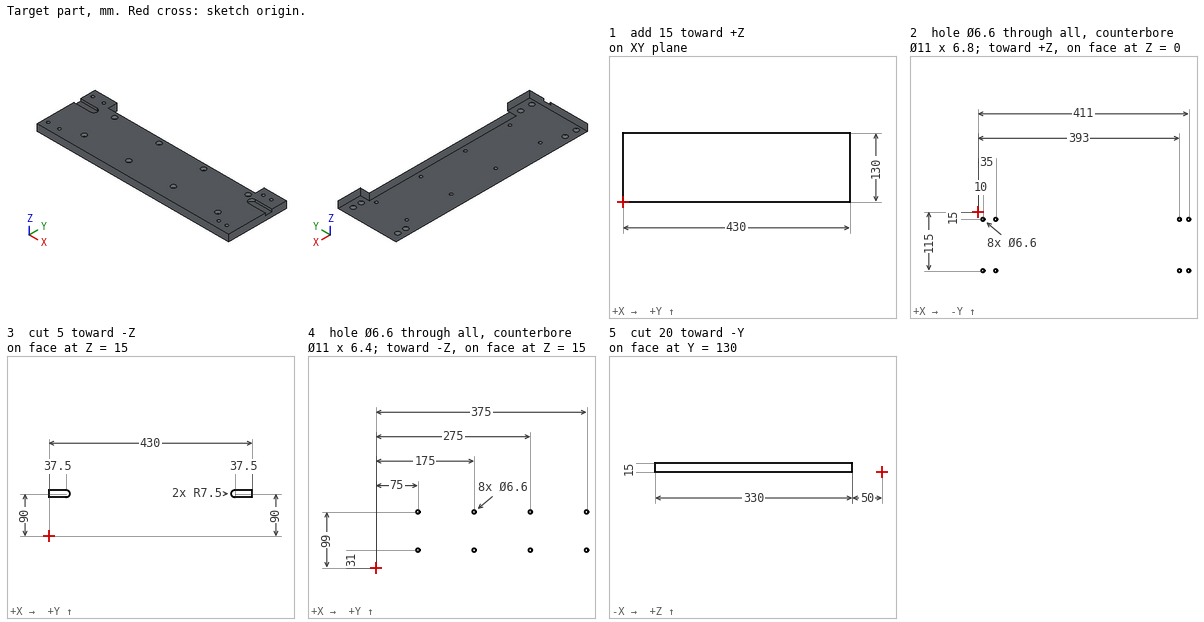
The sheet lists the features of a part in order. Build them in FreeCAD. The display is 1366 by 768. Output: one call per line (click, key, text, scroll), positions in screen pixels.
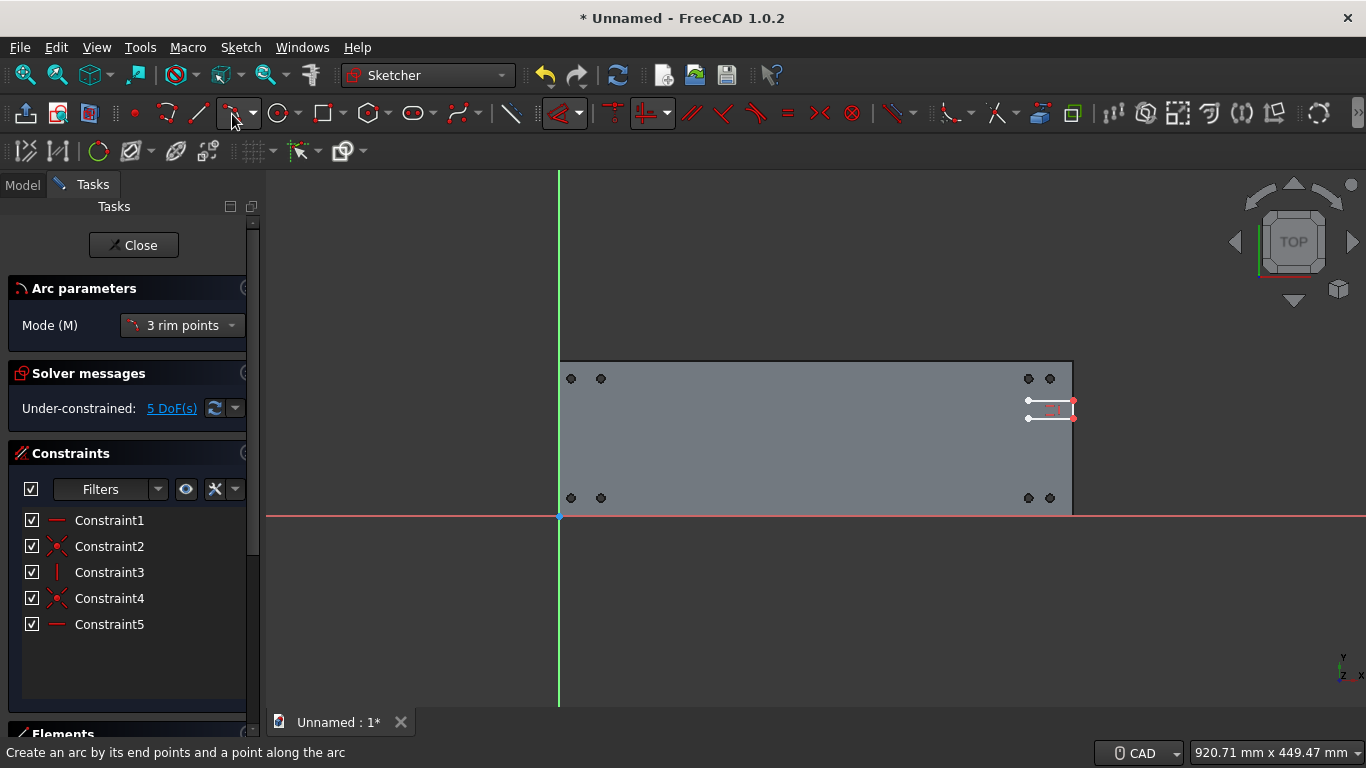
click(1028, 401)
click(1028, 419)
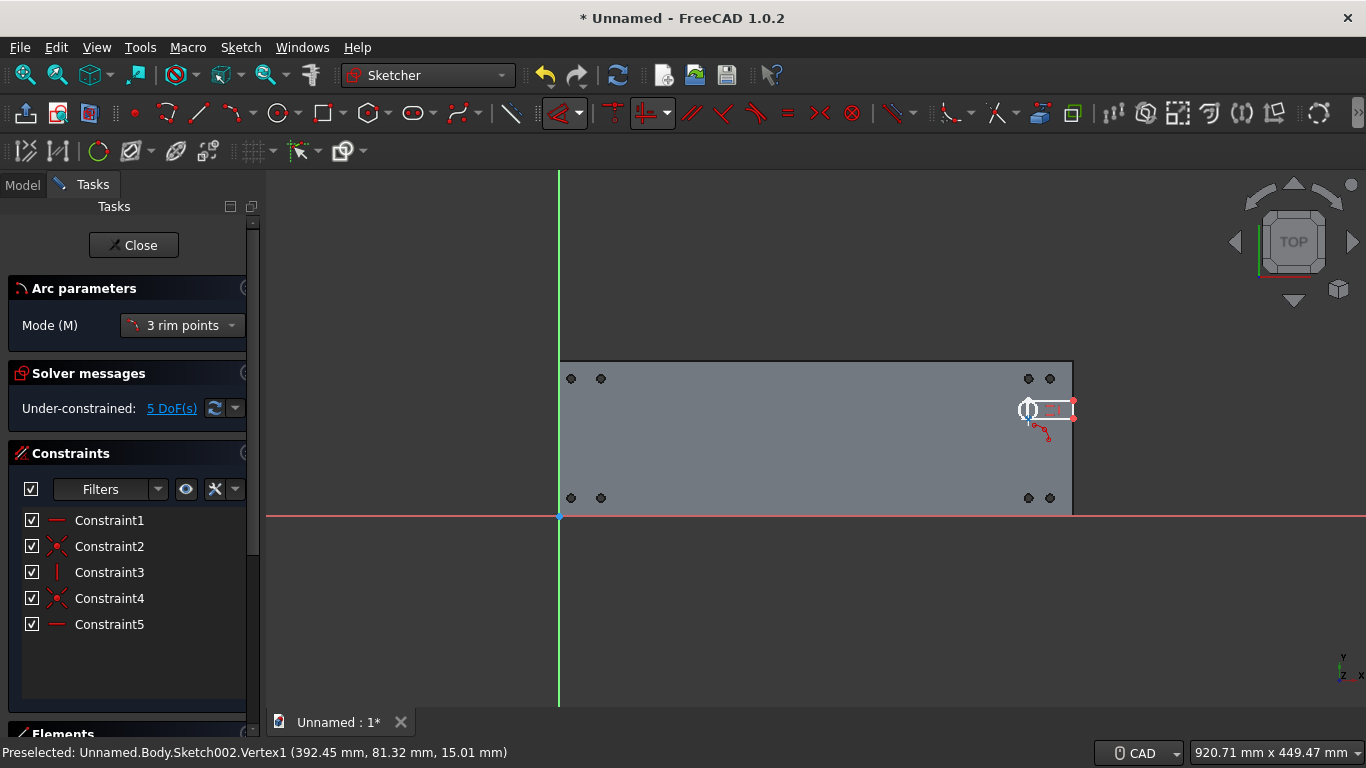
scroll(1019, 409, up, 3)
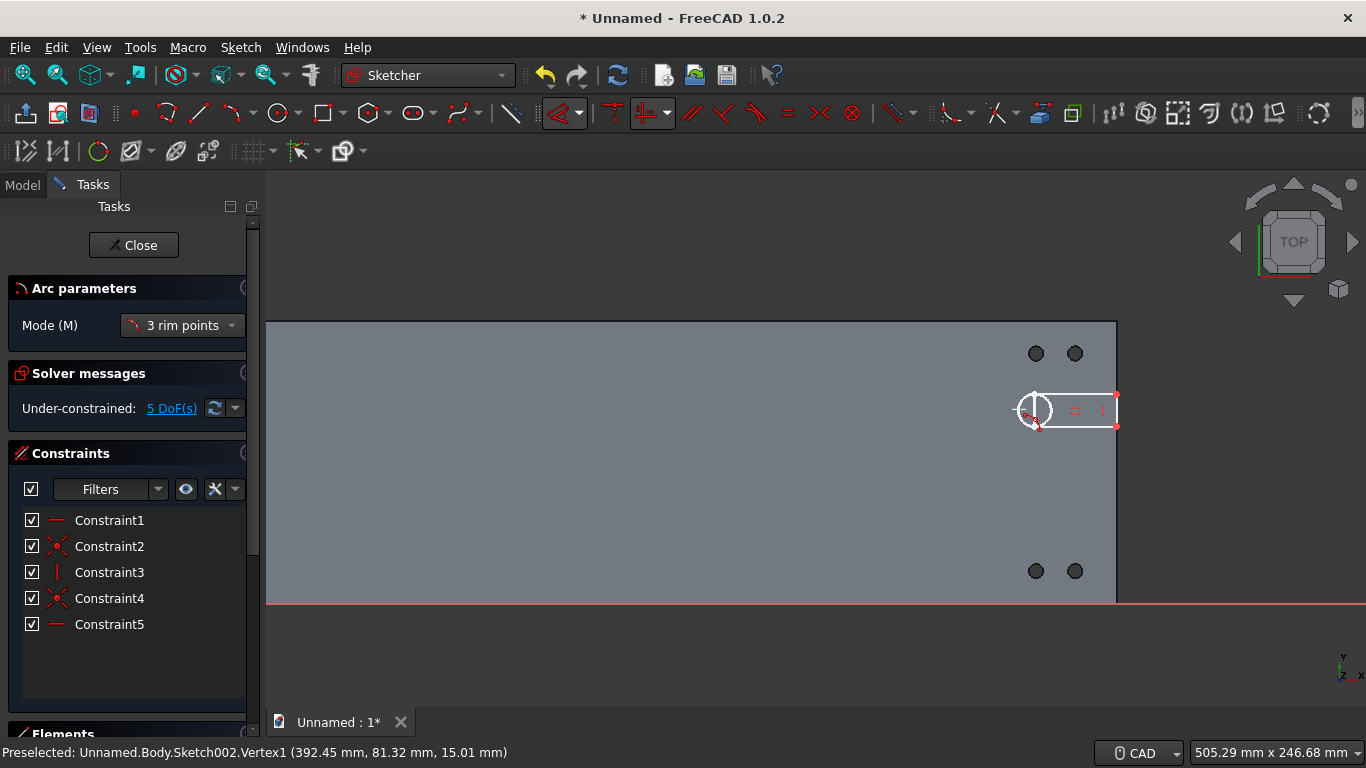
click(1019, 408)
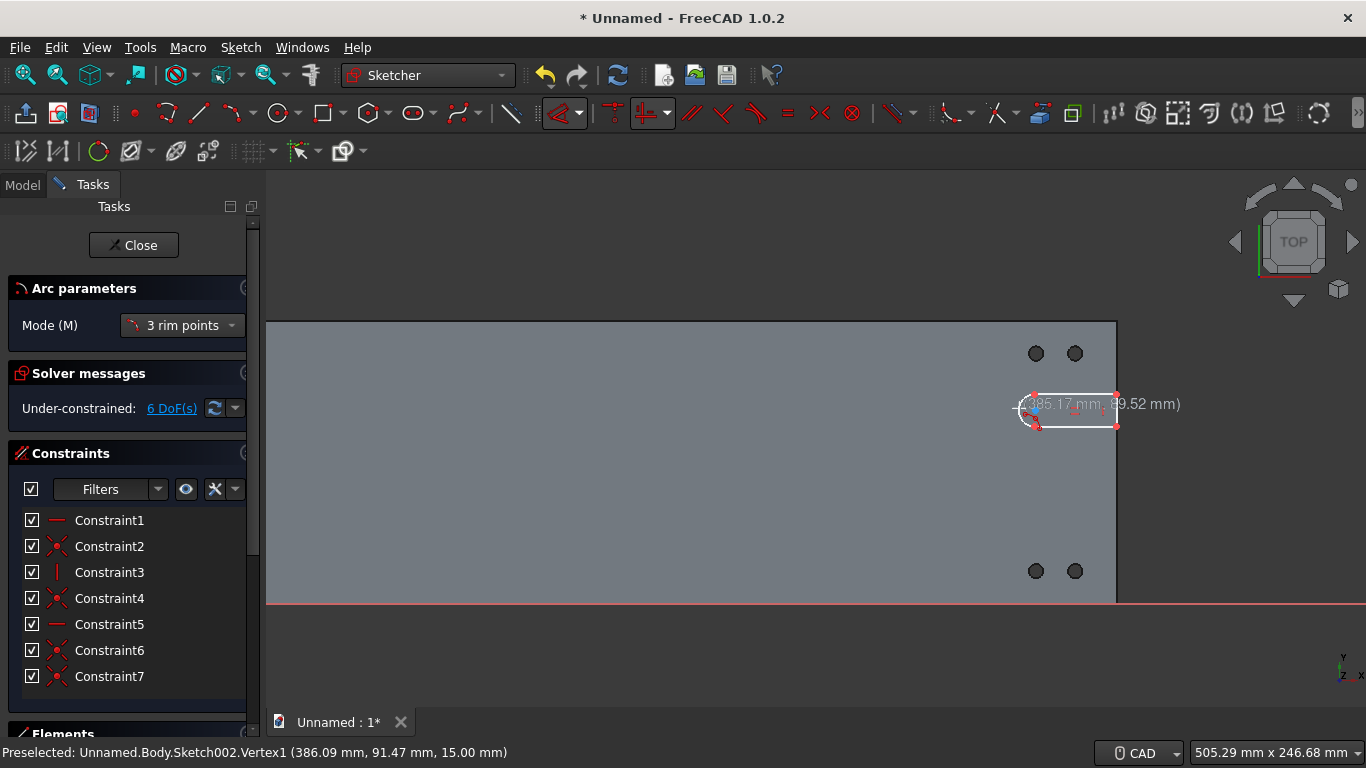
click(168, 114)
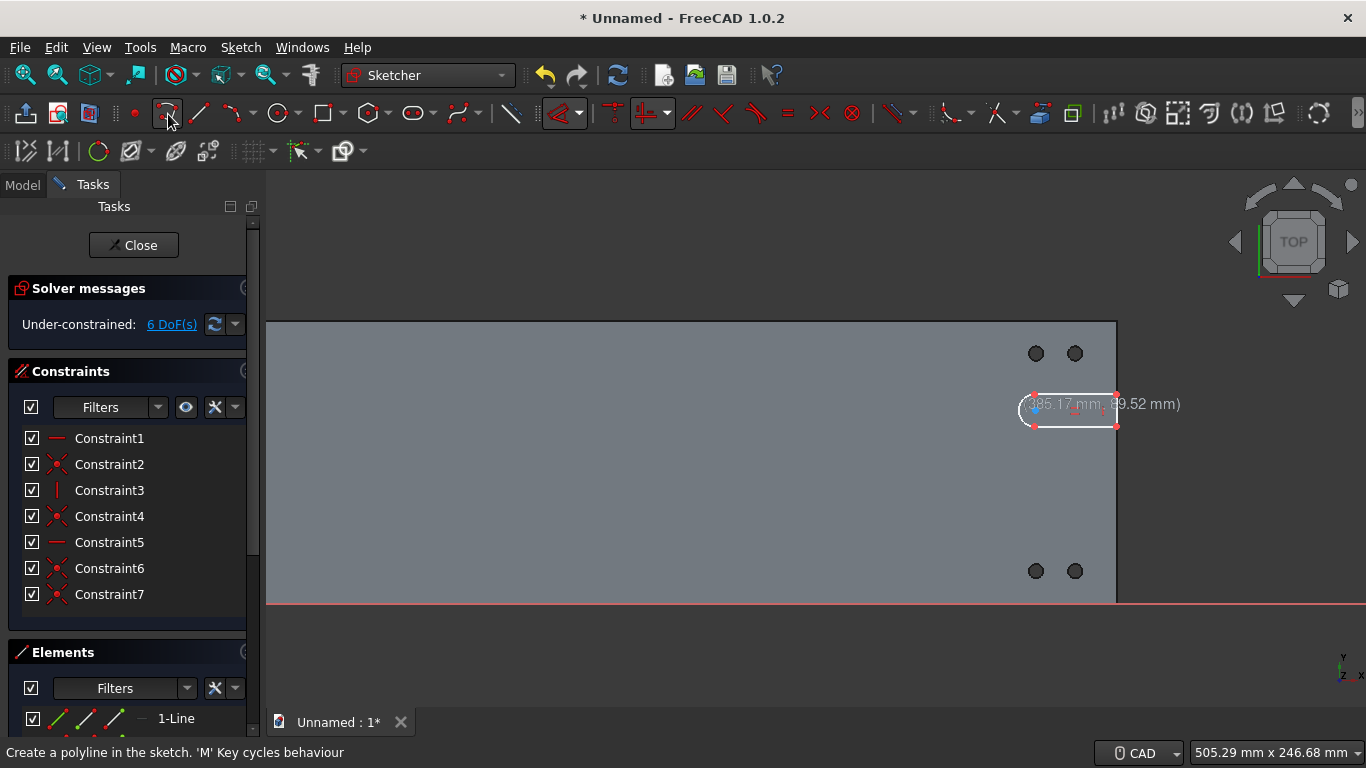
scroll(949, 318, down, 2)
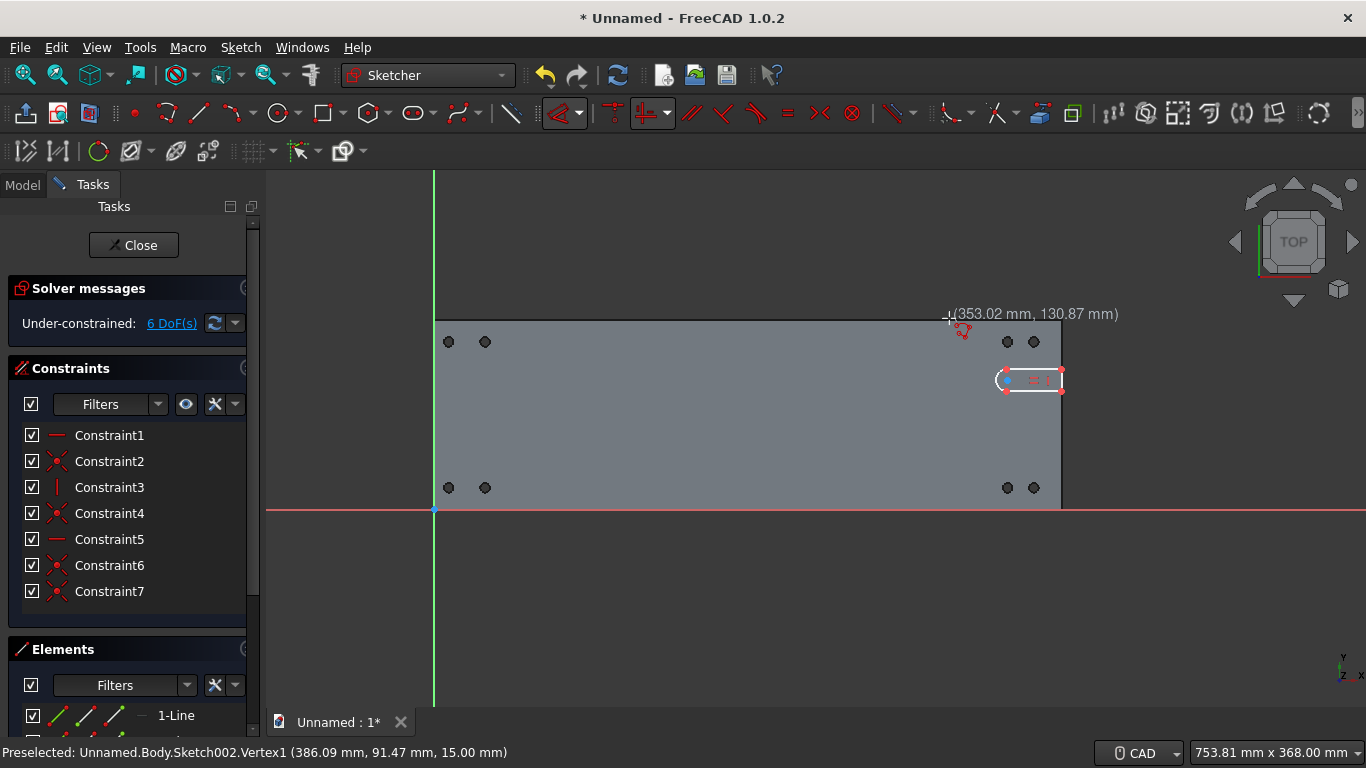
click(489, 367)
click(434, 367)
click(443, 389)
click(489, 389)
right_click(489, 389)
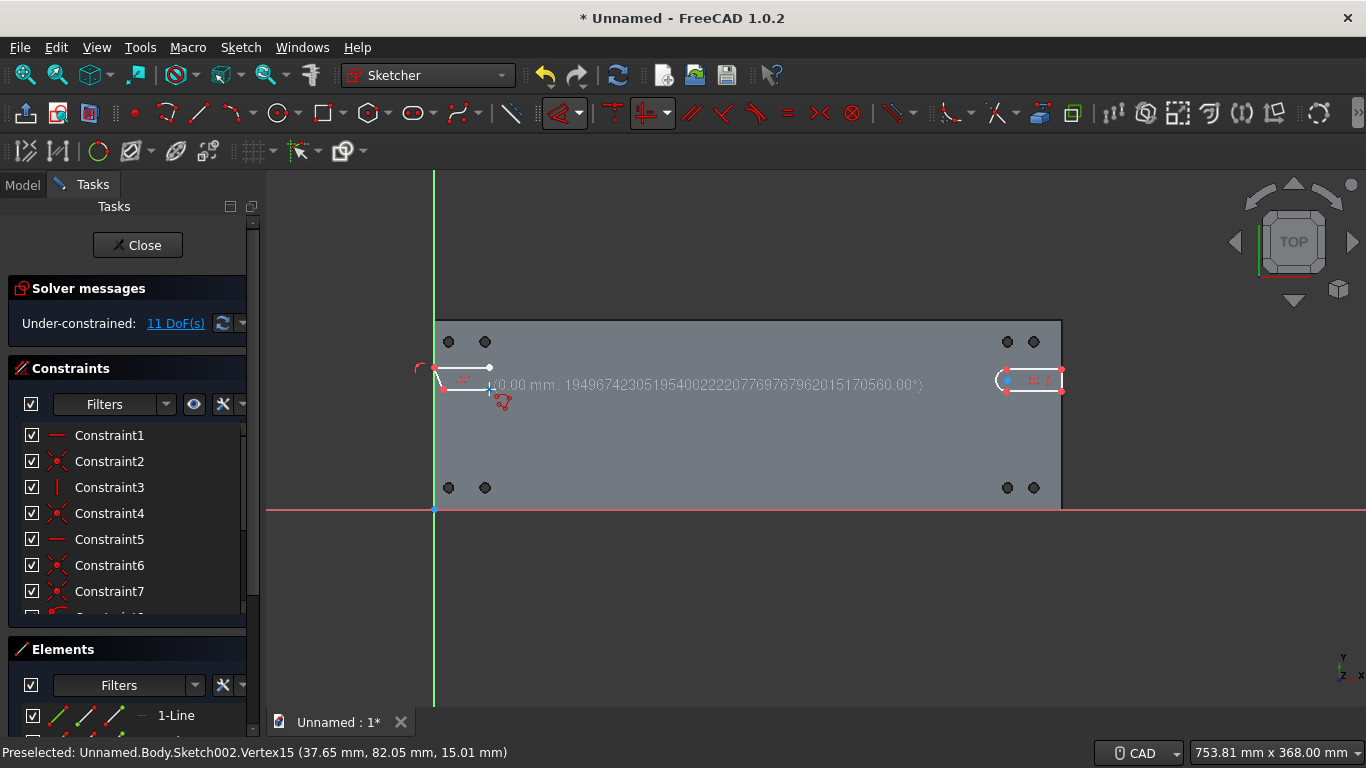
key(g)
key(3)
key(a)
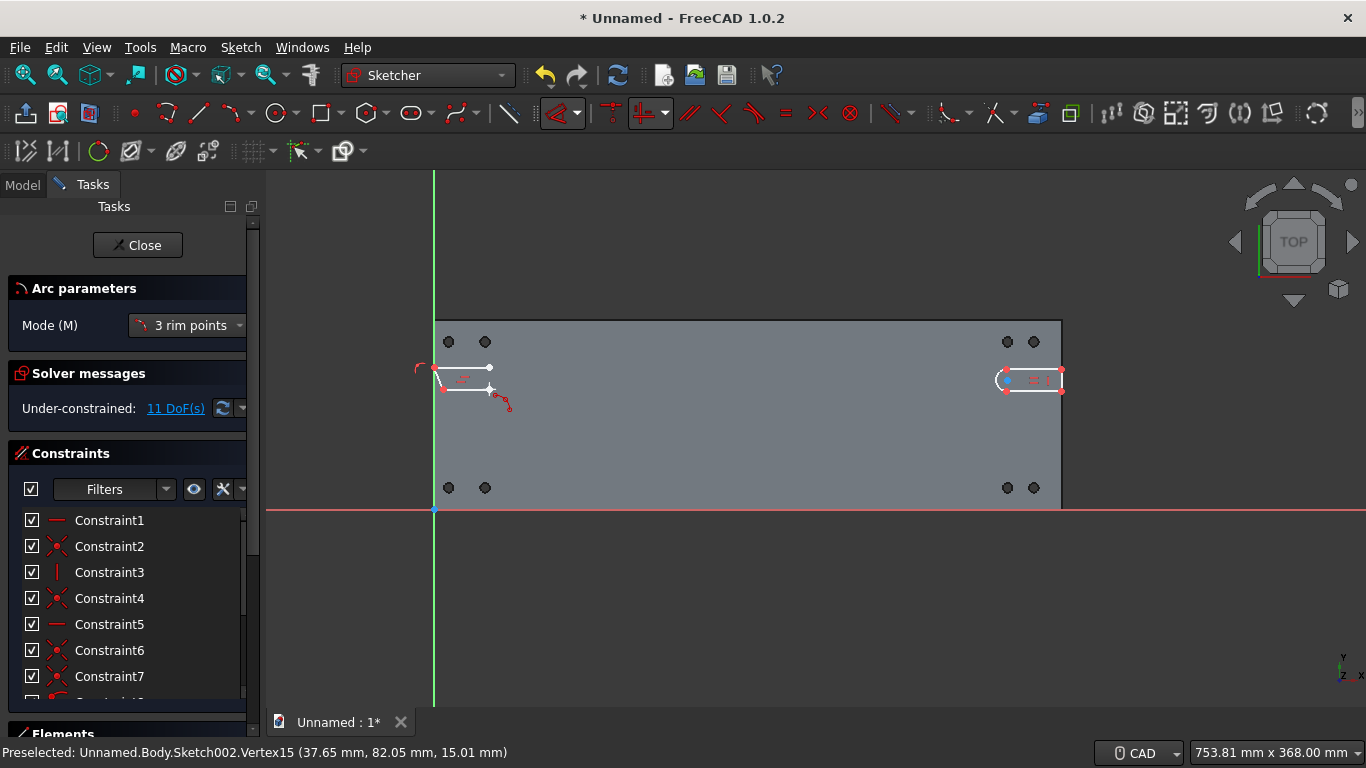
click(489, 390)
click(489, 368)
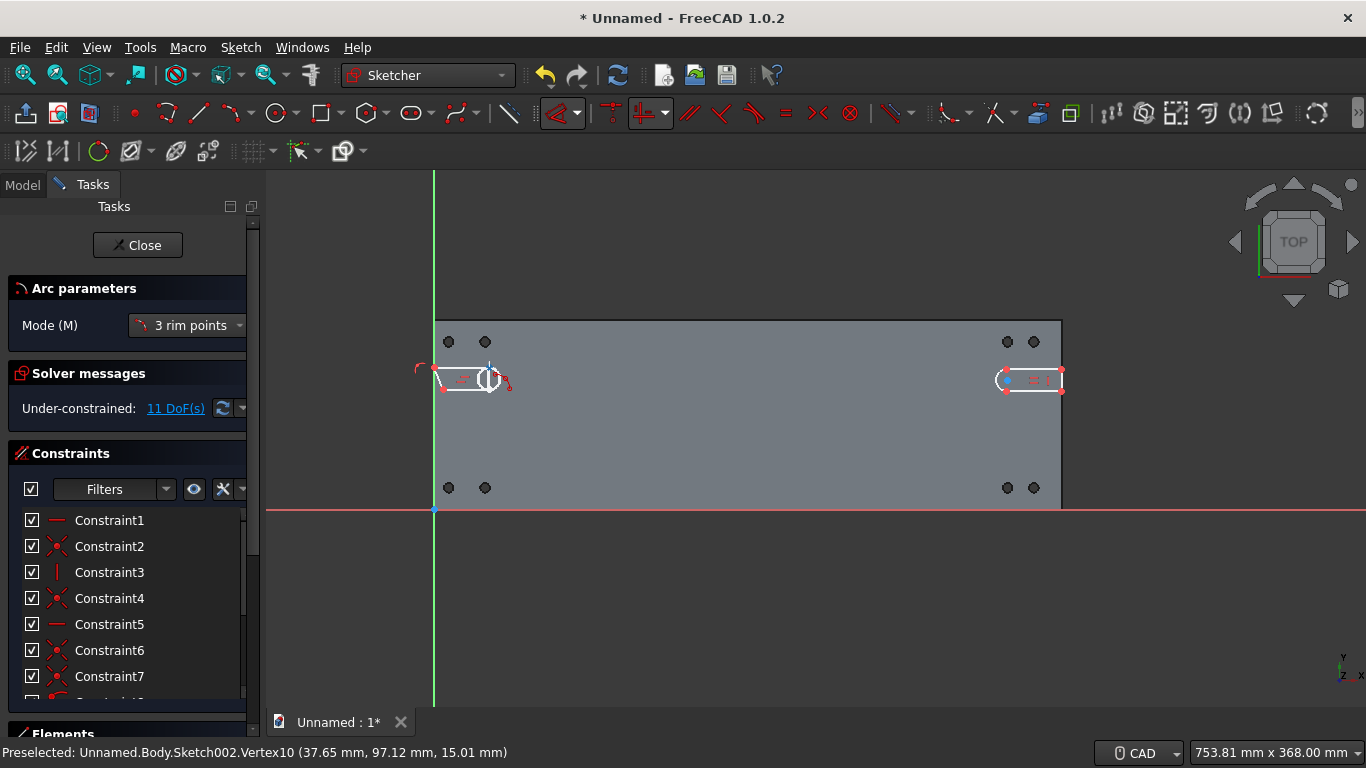
scroll(500, 378, up, 2)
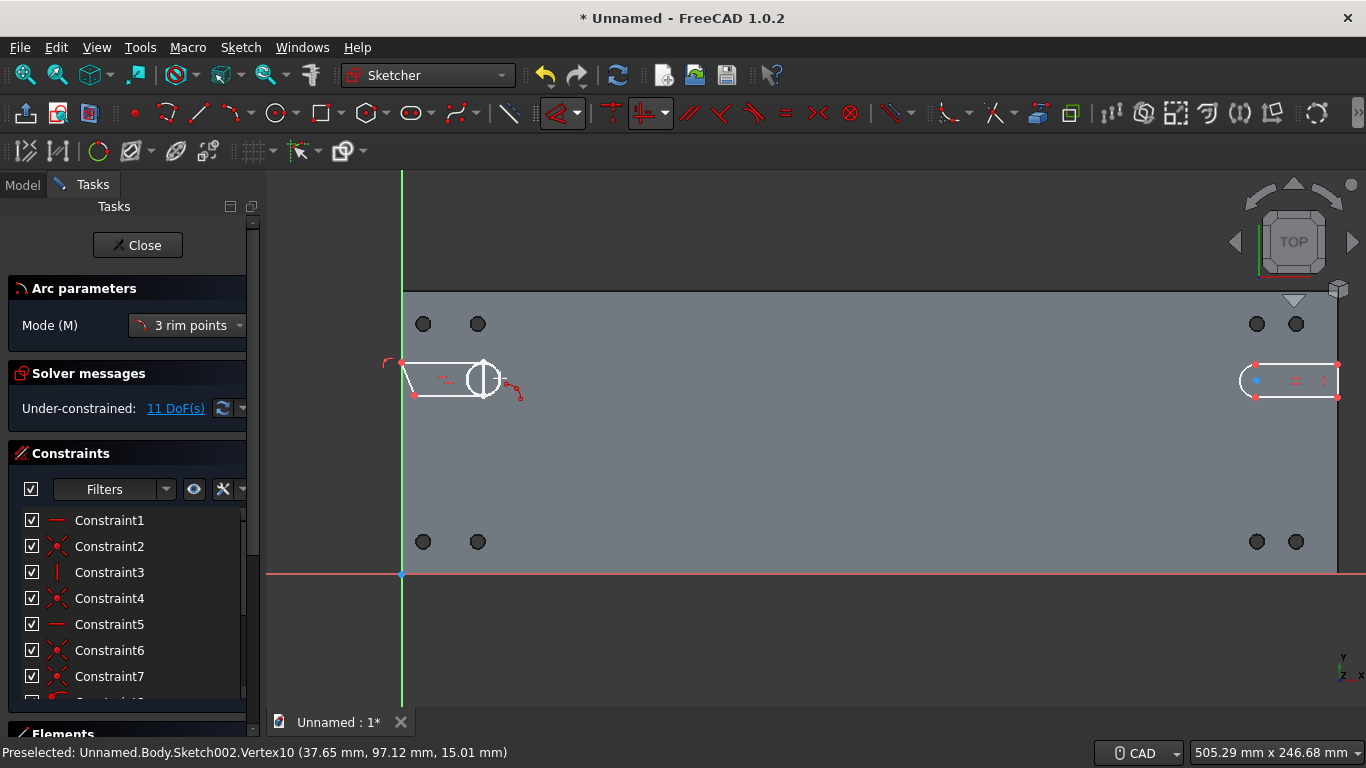
click(499, 378)
key(Escape)